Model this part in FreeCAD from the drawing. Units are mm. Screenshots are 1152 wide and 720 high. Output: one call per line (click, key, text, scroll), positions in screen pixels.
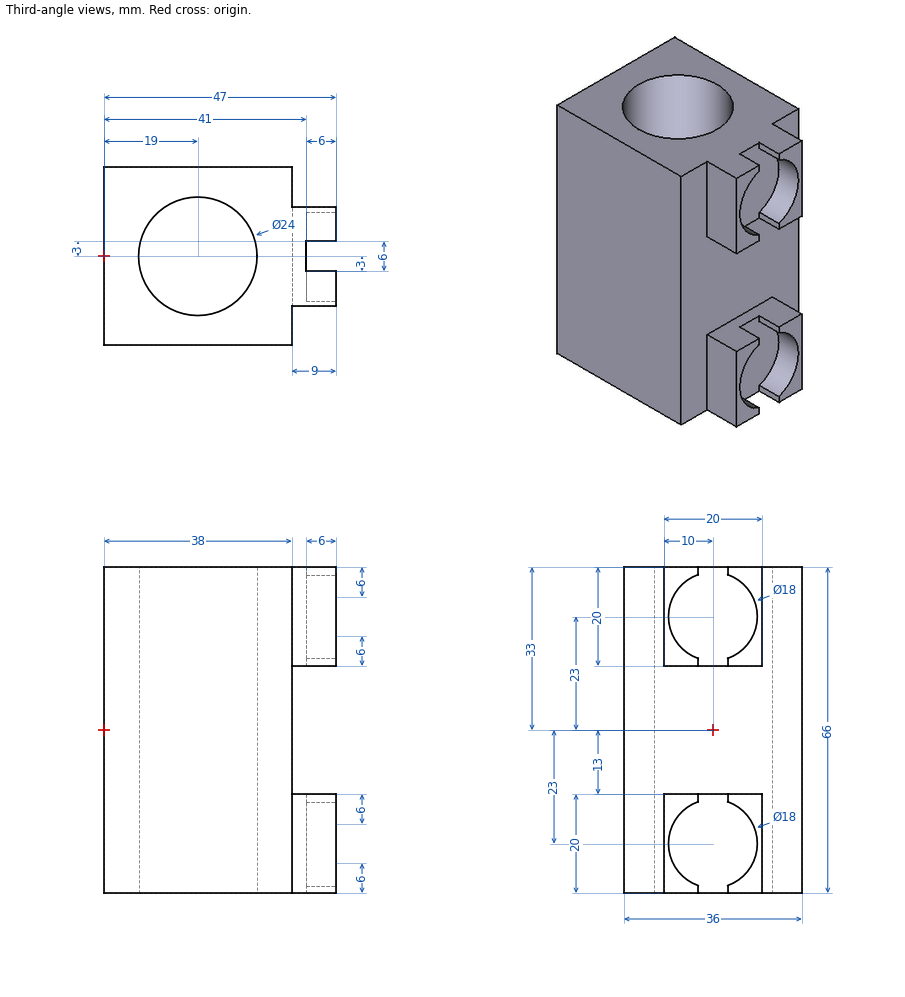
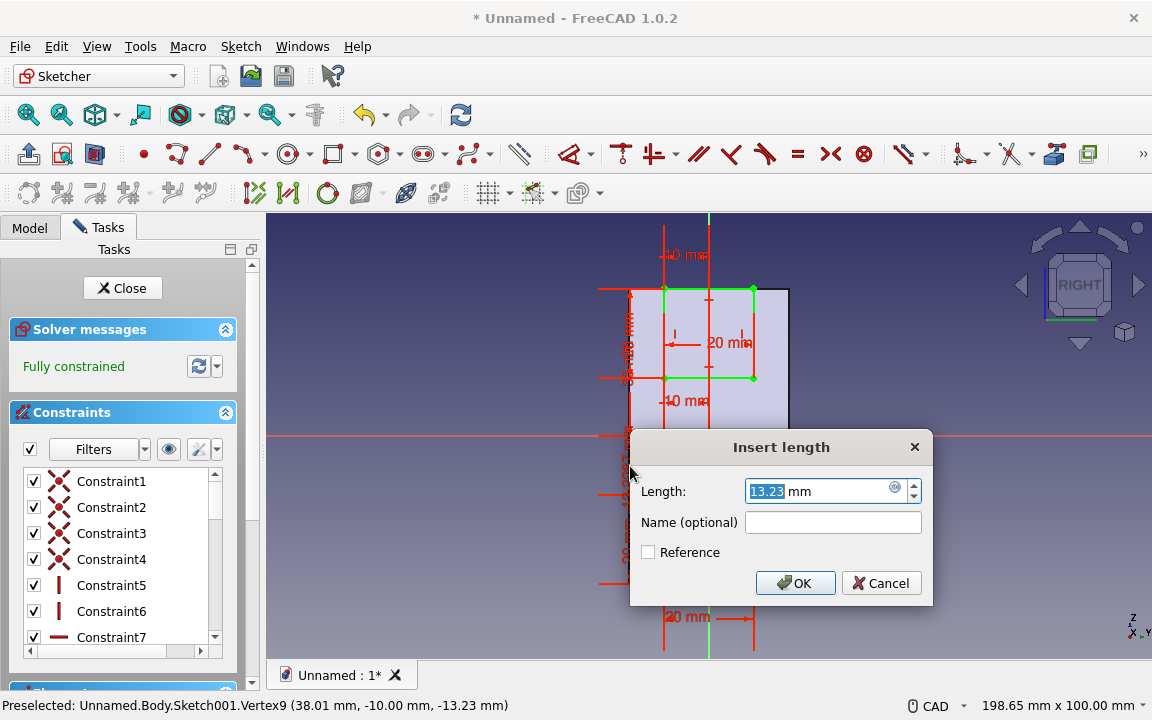
text(13)
key(Return)
key(Escape)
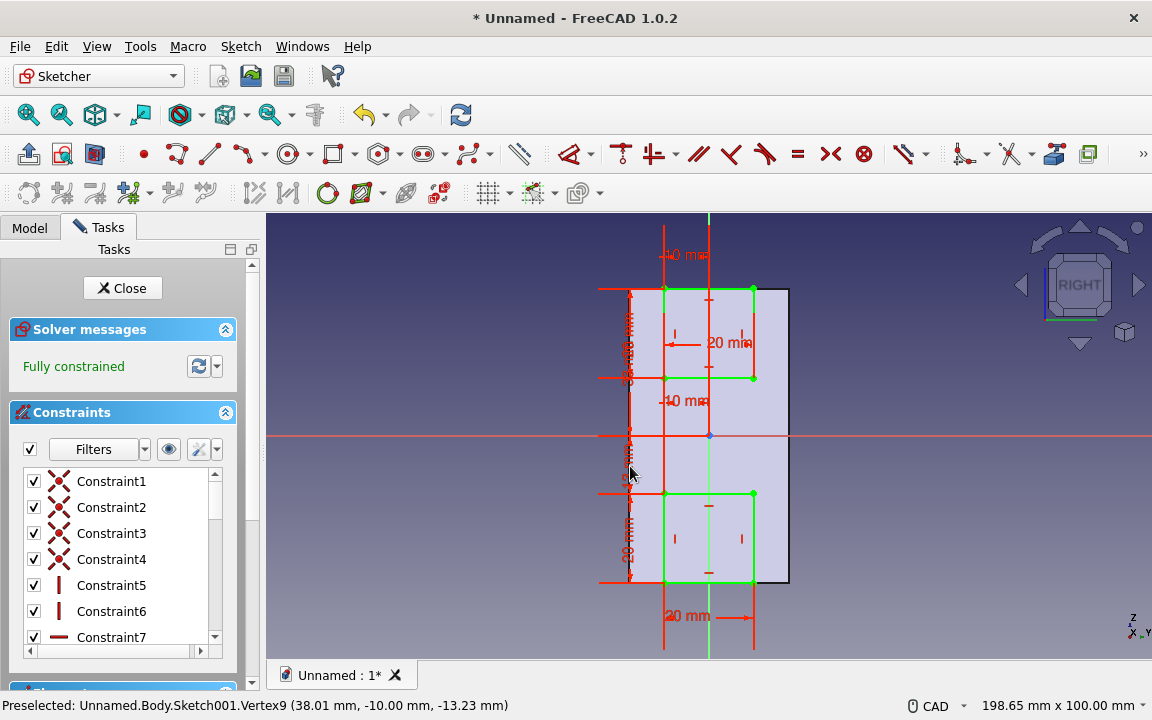
click(123, 288)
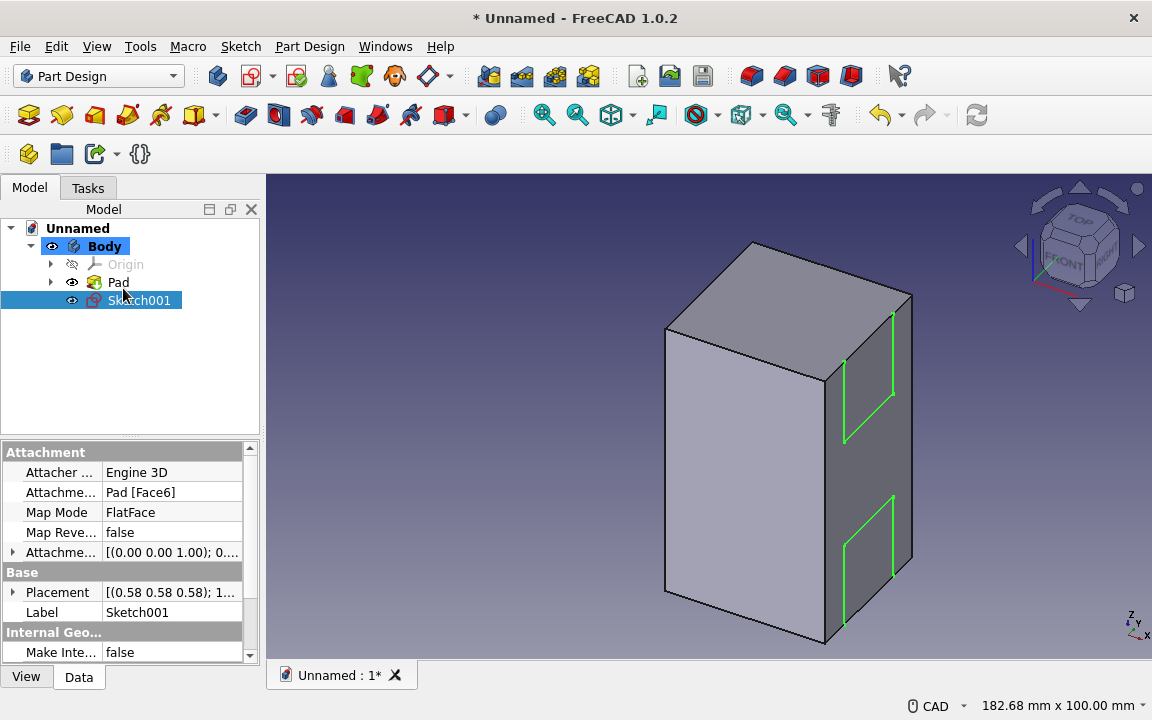
click(29, 116)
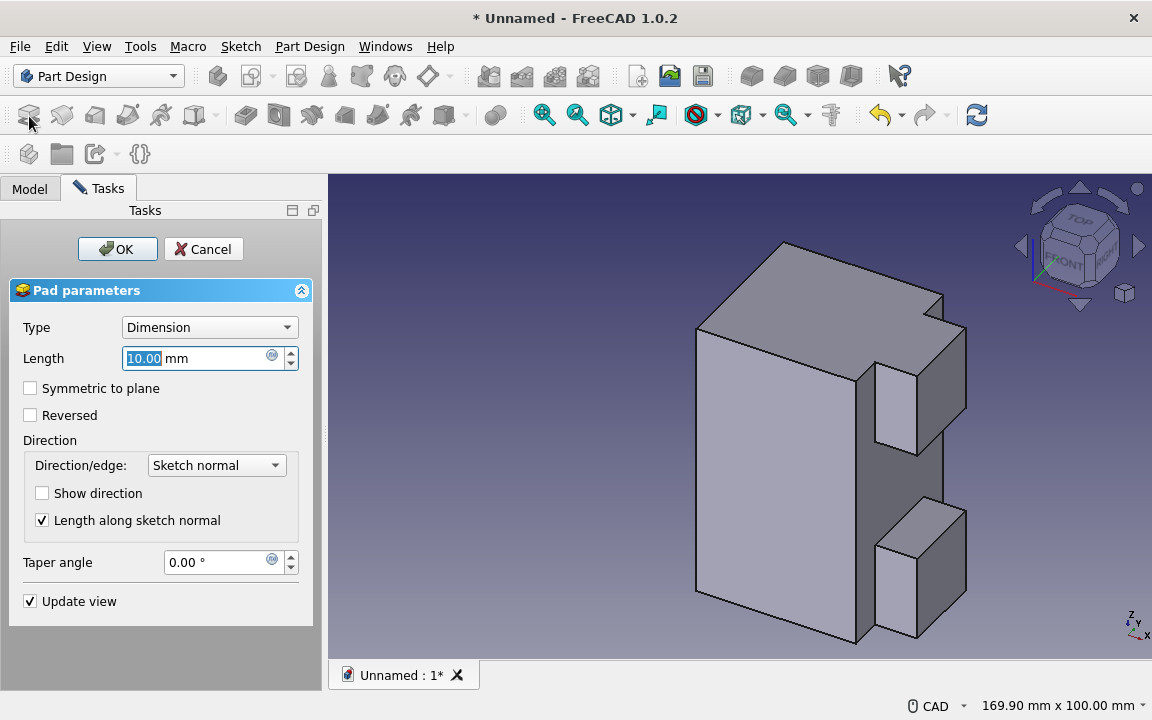
text(9)
key(Tab)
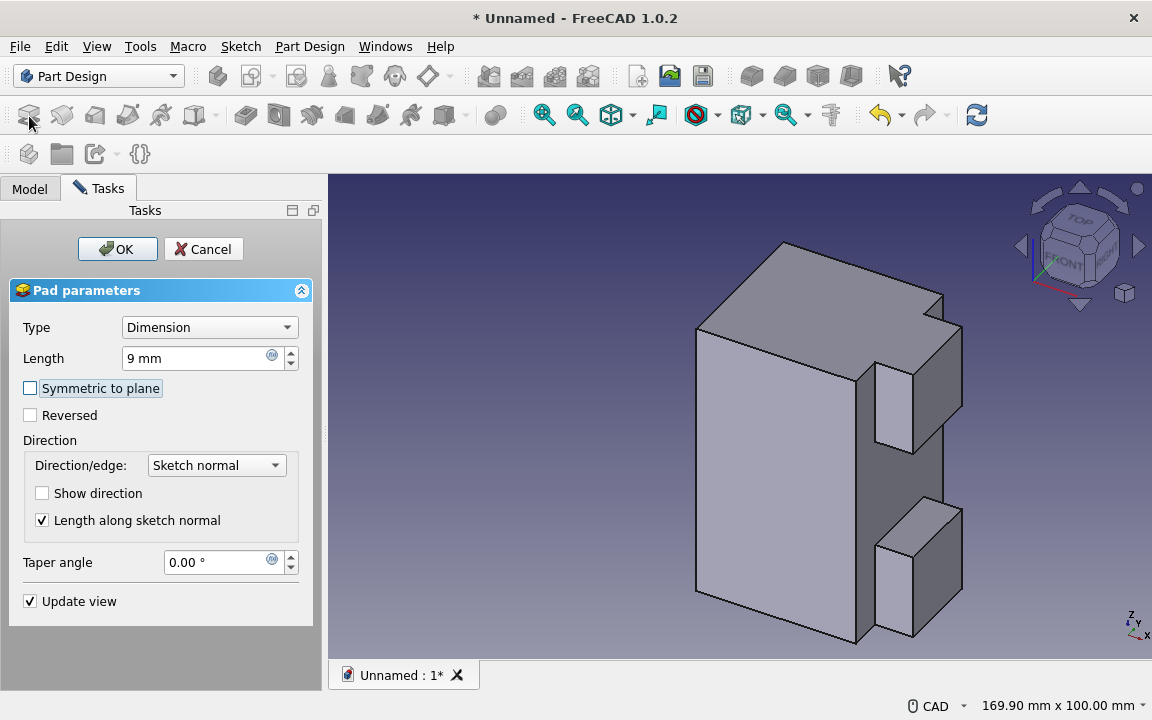
click(118, 249)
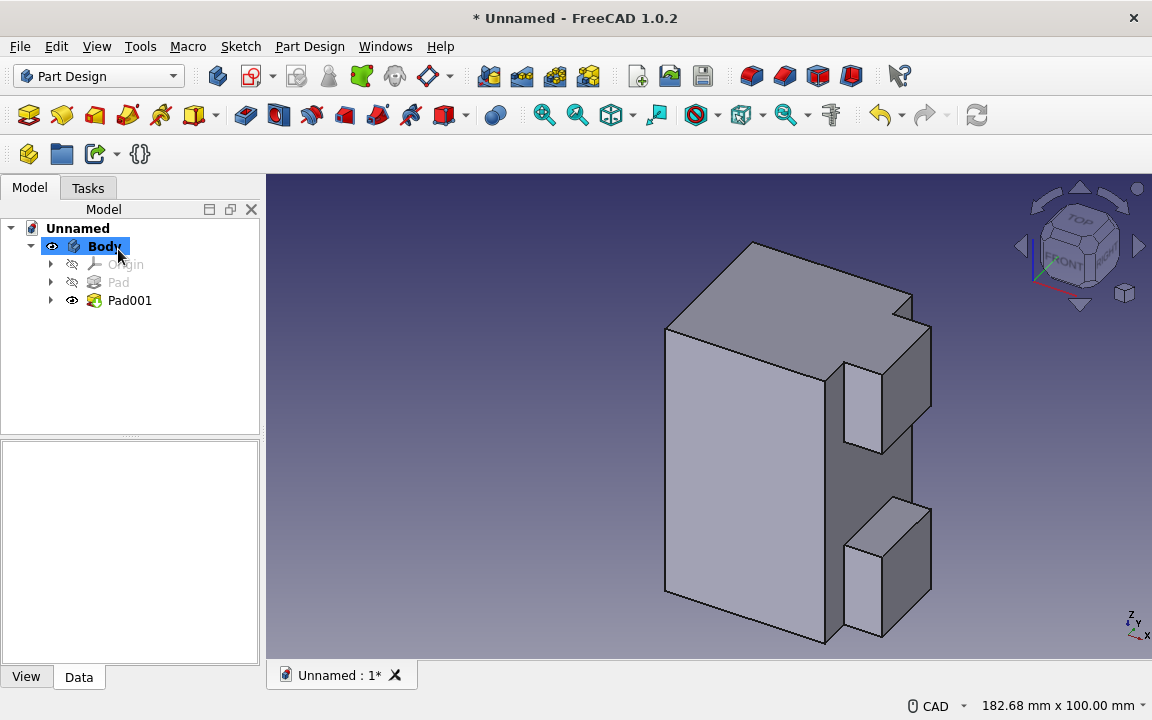
click(906, 389)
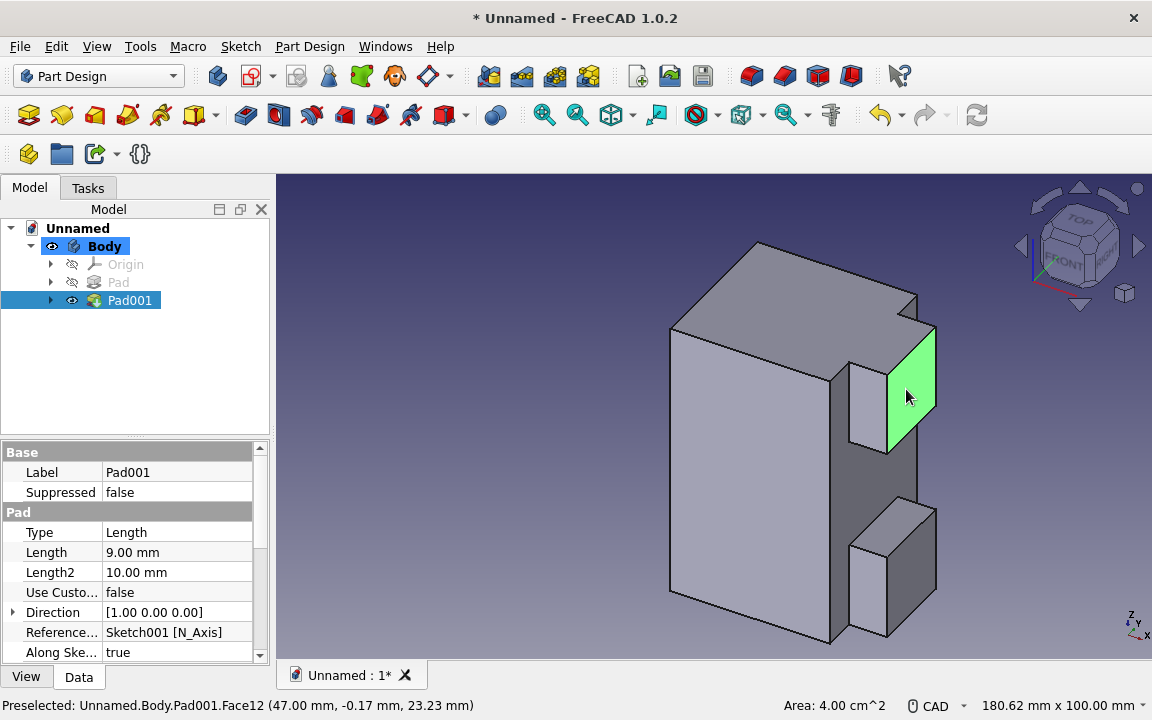
click(250, 76)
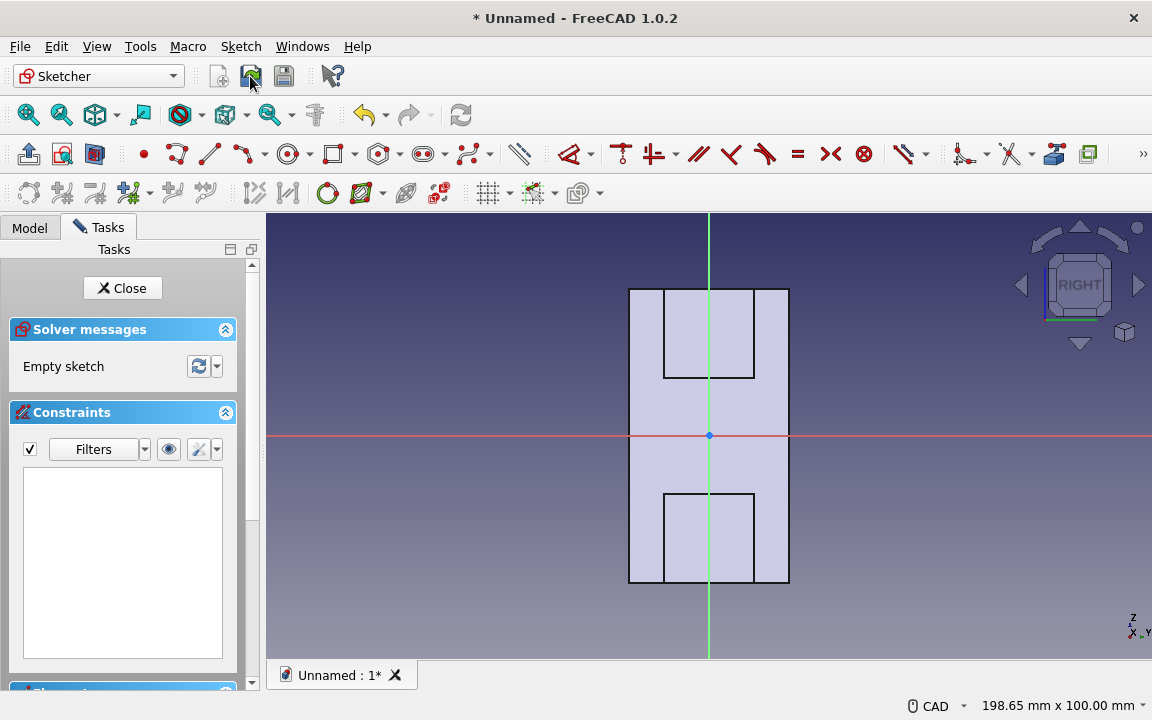
scroll(792, 278, up, 3)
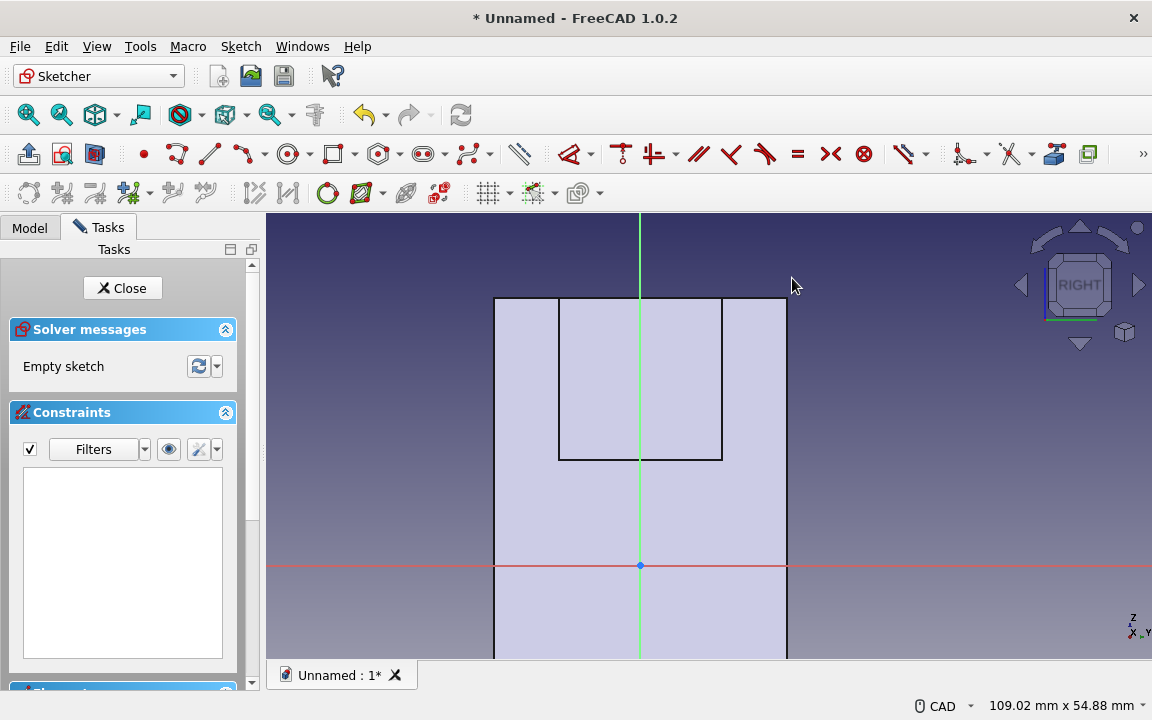
click(288, 154)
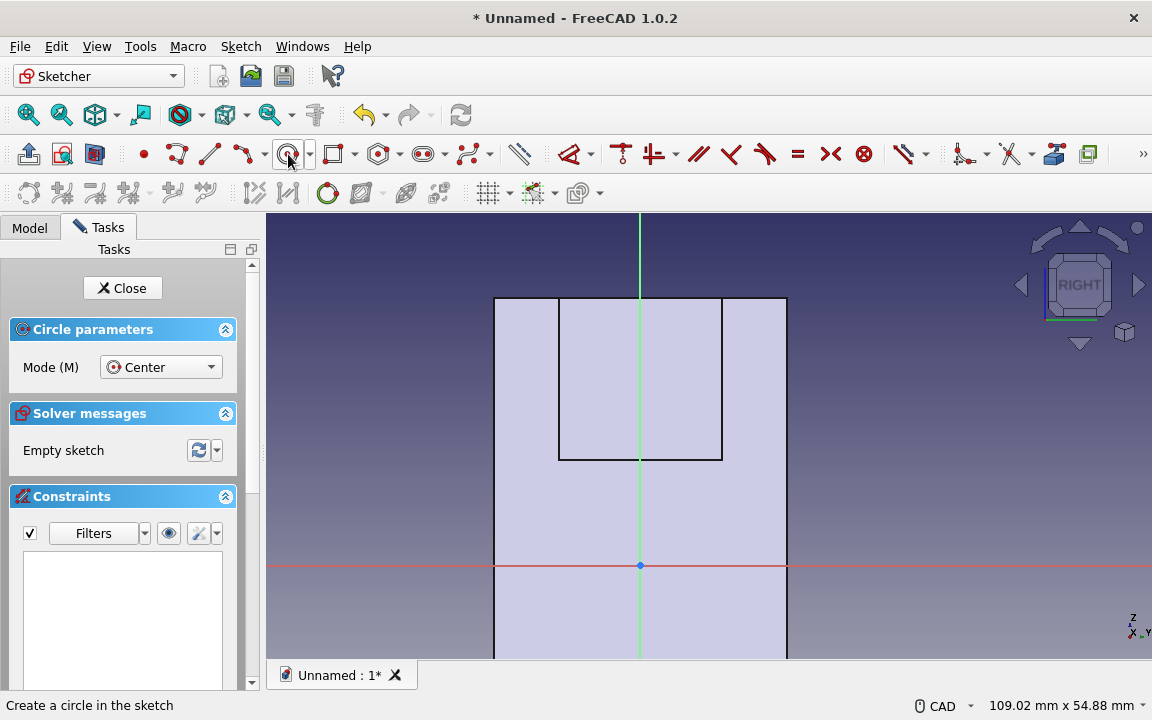
click(640, 379)
click(692, 327)
key(Escape)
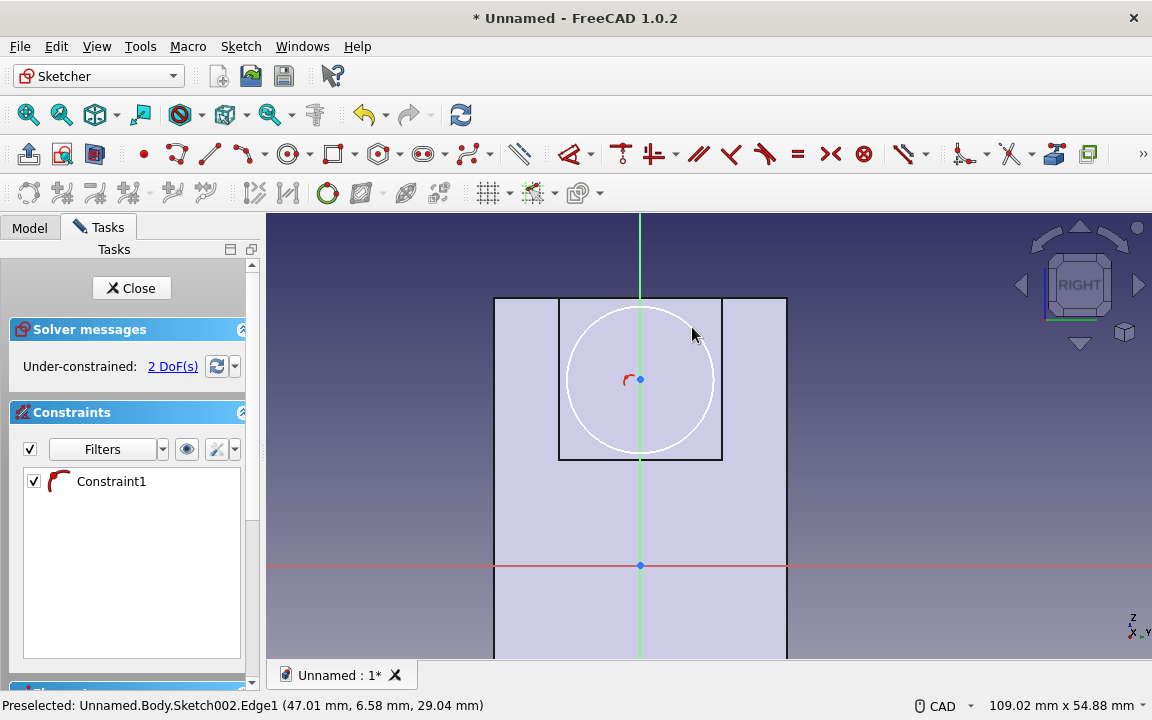
click(568, 154)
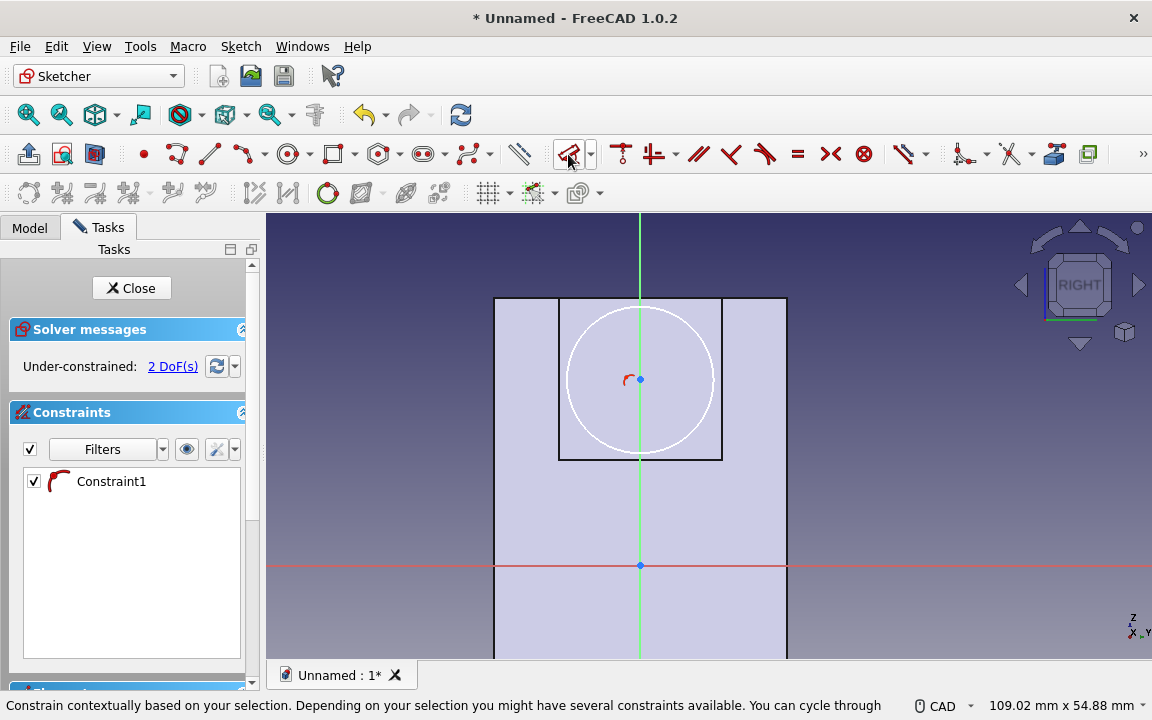
click(692, 328)
click(715, 305)